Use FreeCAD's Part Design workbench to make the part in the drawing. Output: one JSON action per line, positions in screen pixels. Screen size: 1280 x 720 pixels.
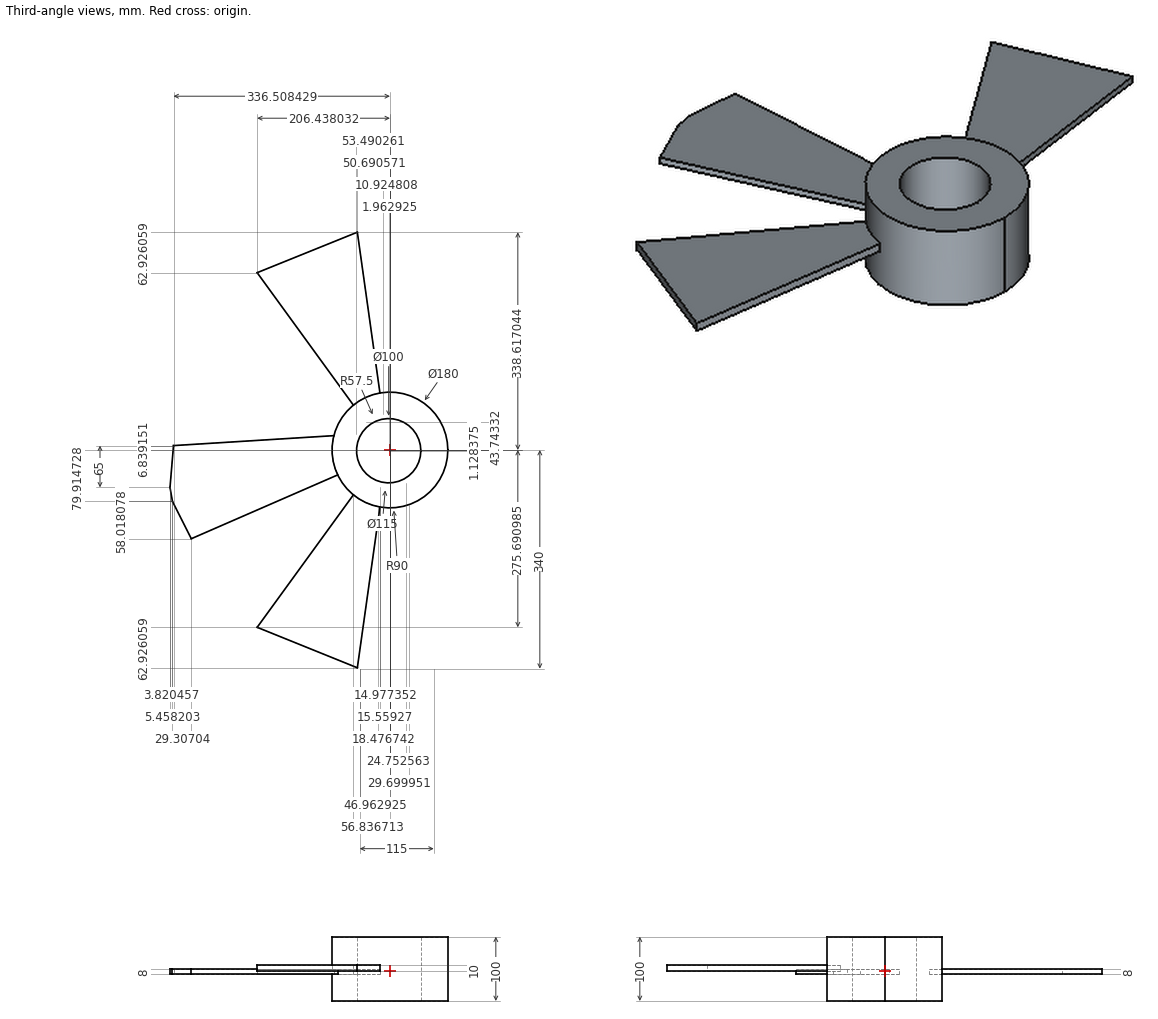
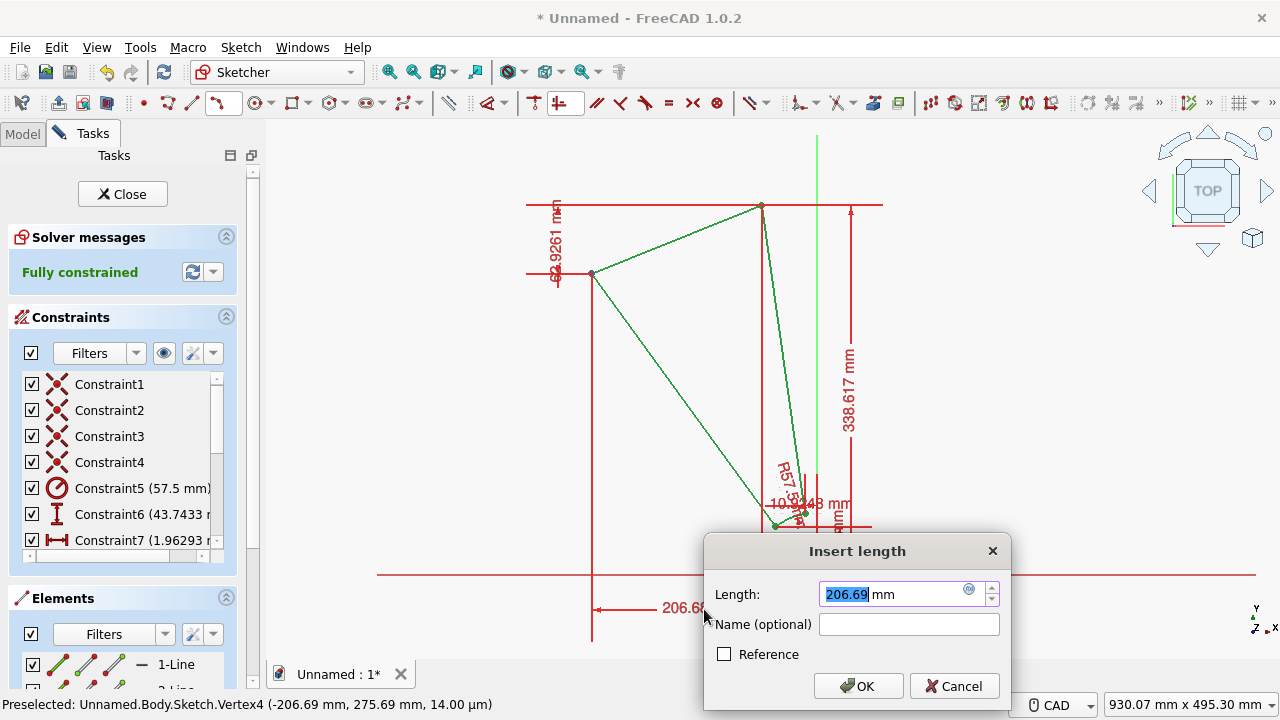
{"action": "type", "text": "206.438032"}
{"action": "key", "text": "Return"}
{"action": "key", "text": "Escape"}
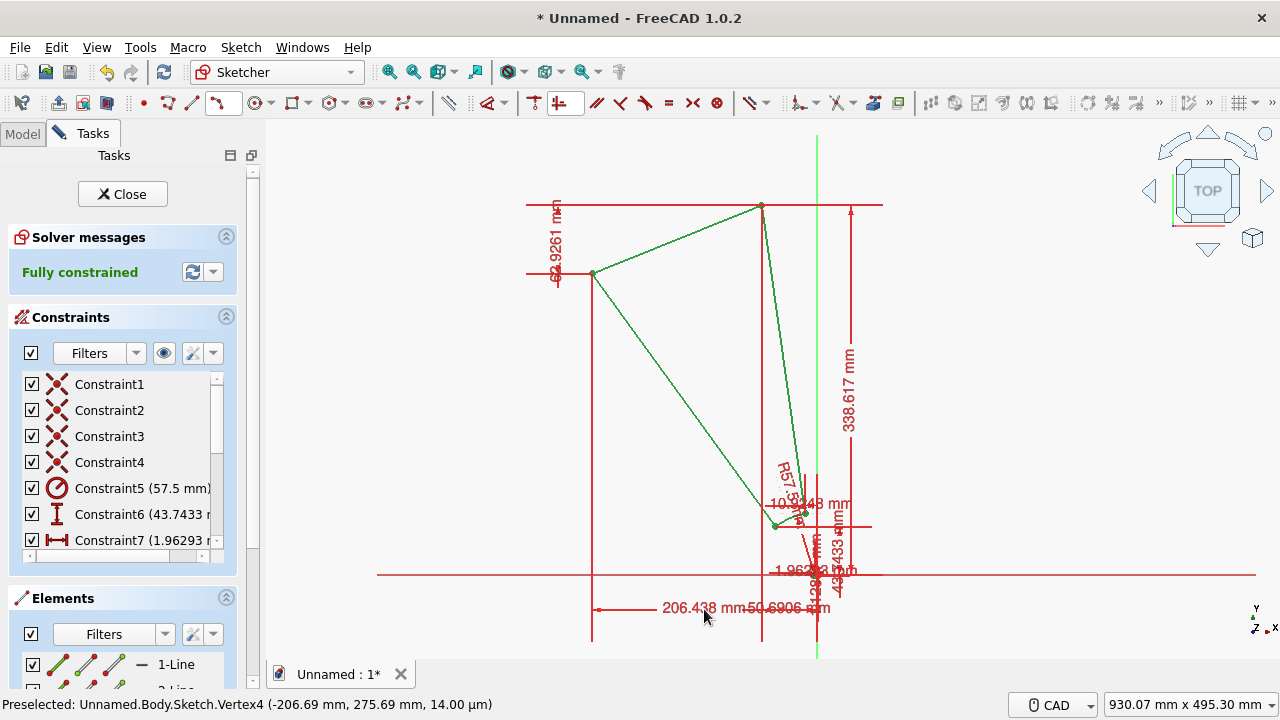
{"action": "left_click", "coordinate": [123, 194]}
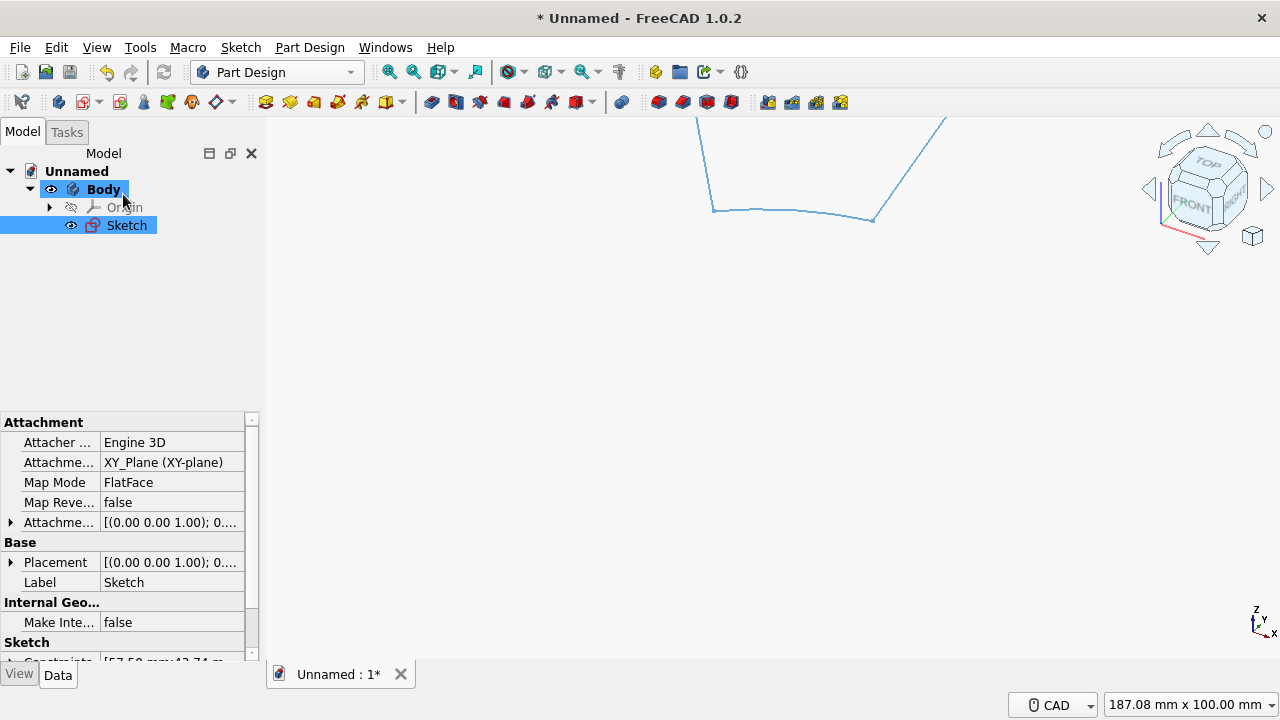
{"action": "left_click", "coordinate": [266, 102]}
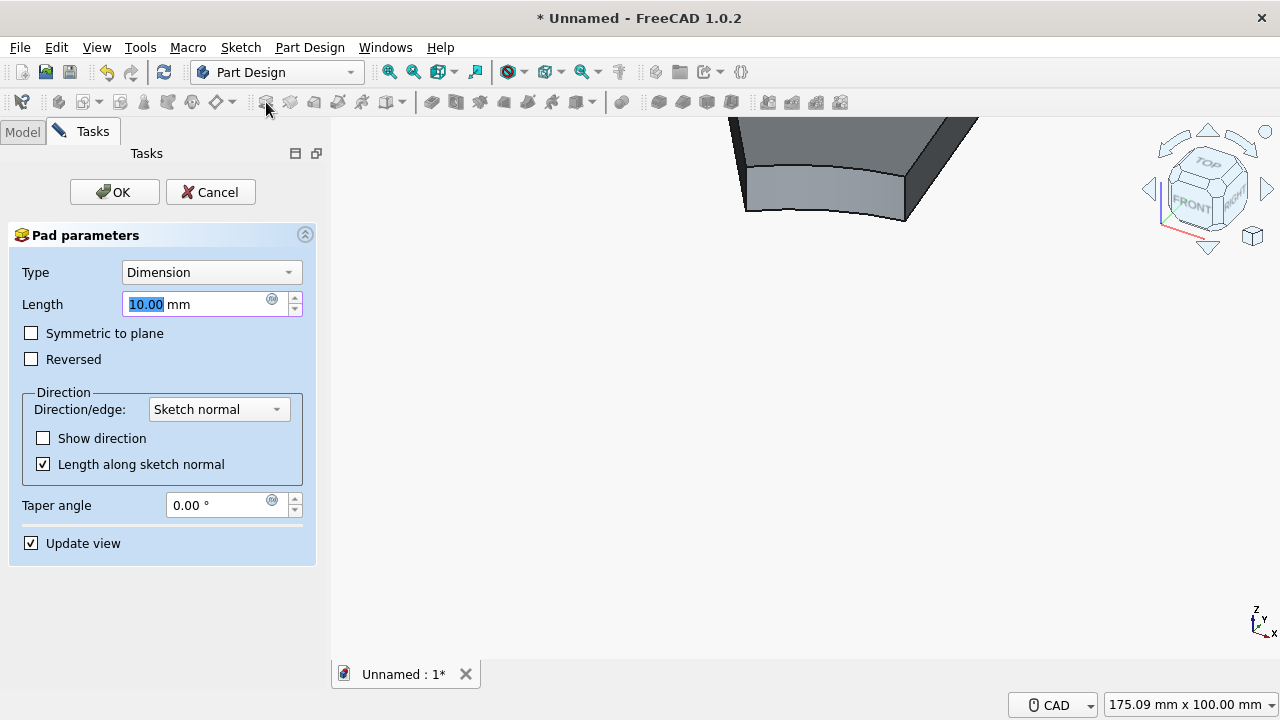
{"action": "type", "text": "8"}
{"action": "key", "text": "Tab"}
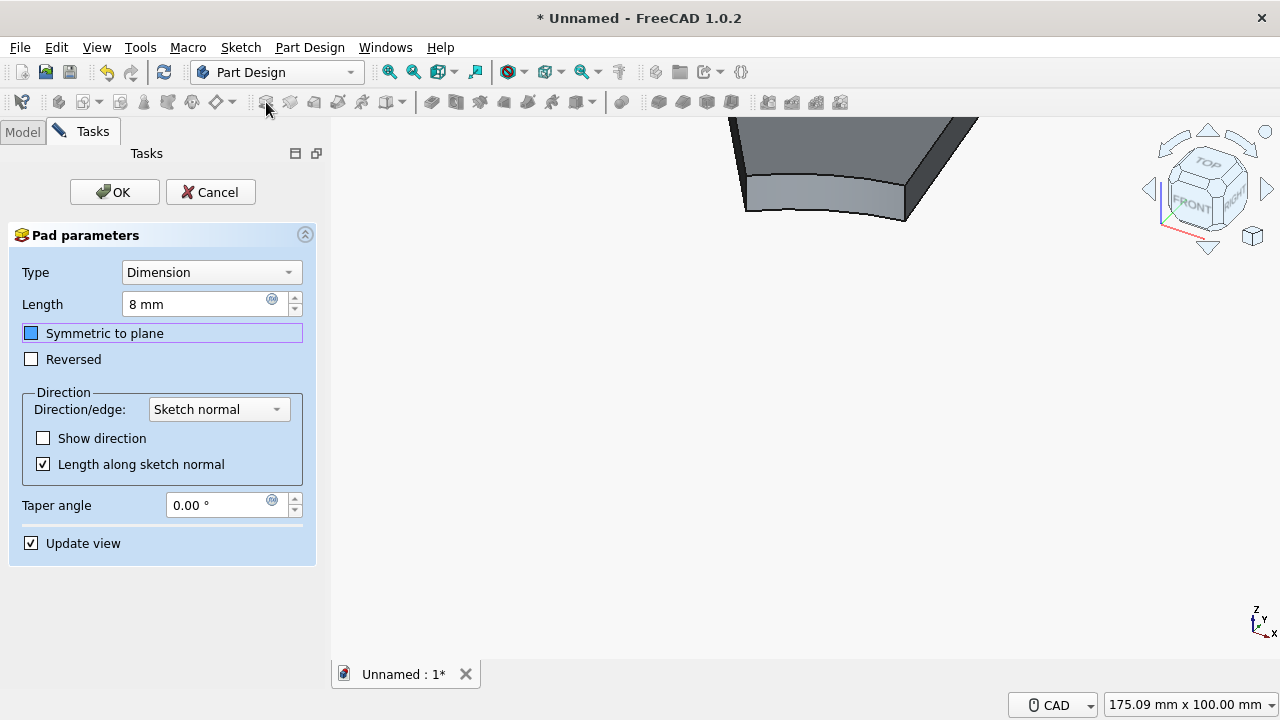
{"action": "left_click", "coordinate": [30, 333]}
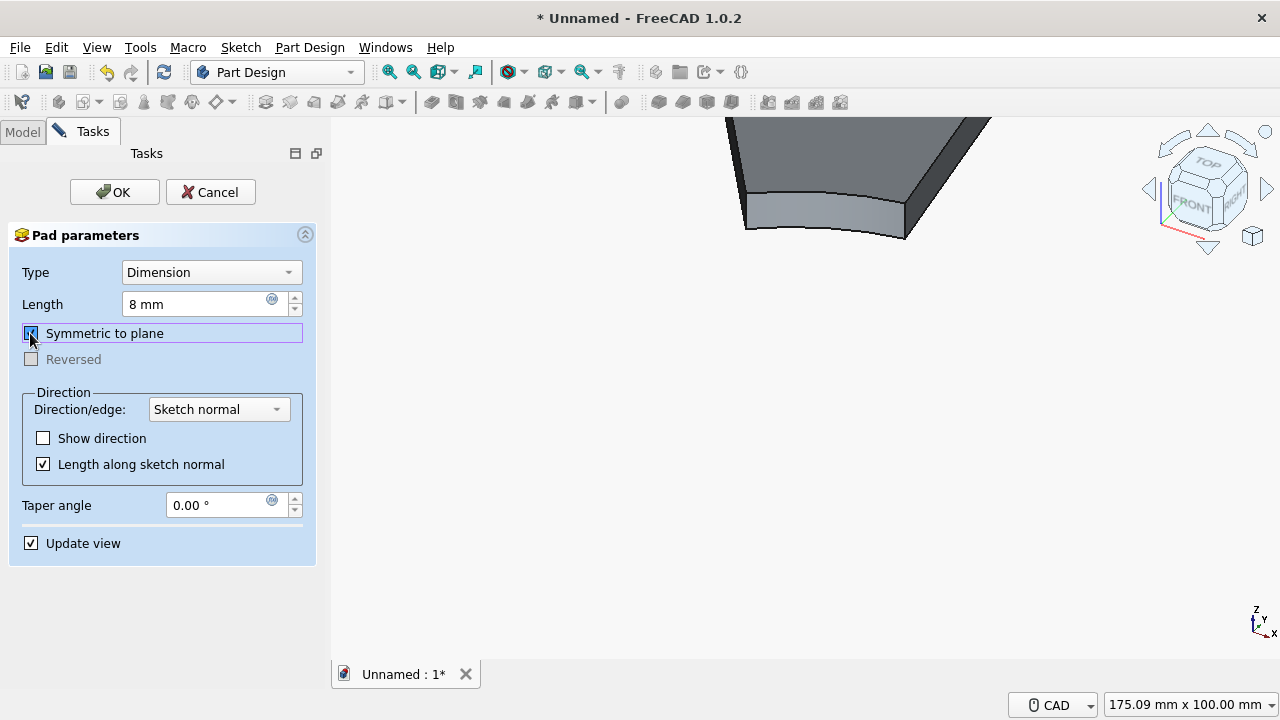
{"action": "left_click", "coordinate": [115, 192]}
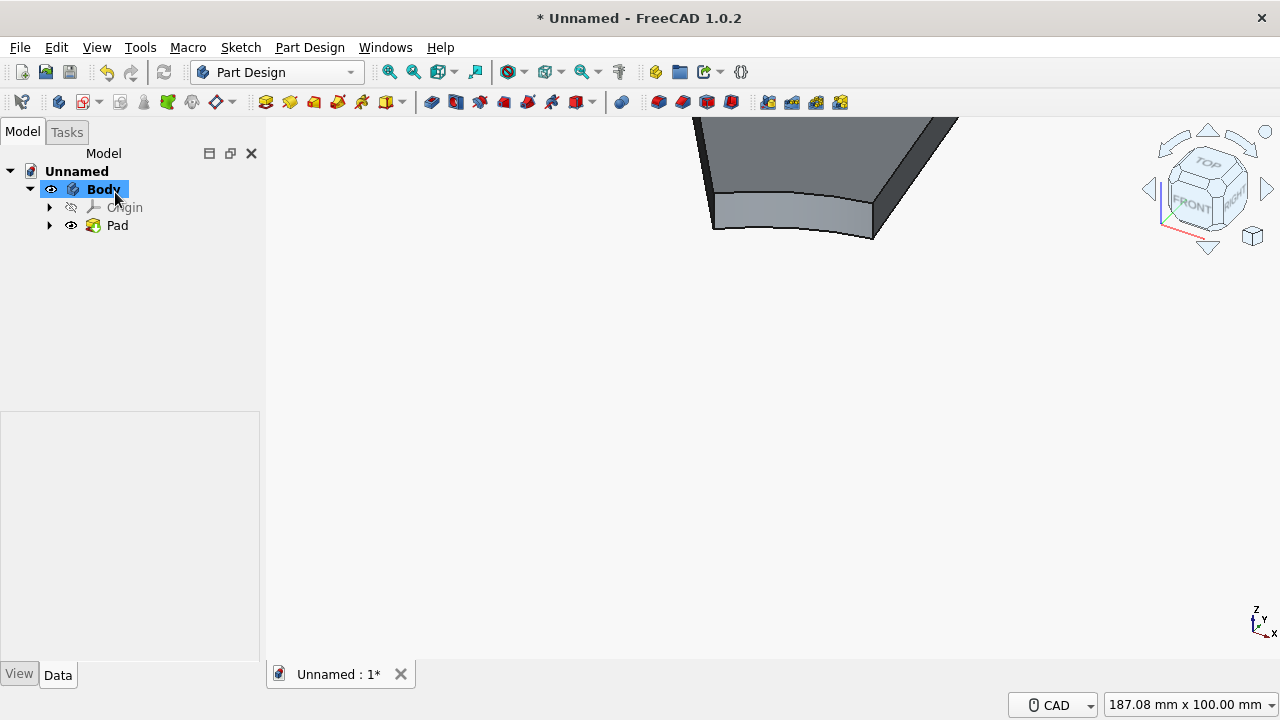
{"action": "left_click", "coordinate": [390, 72]}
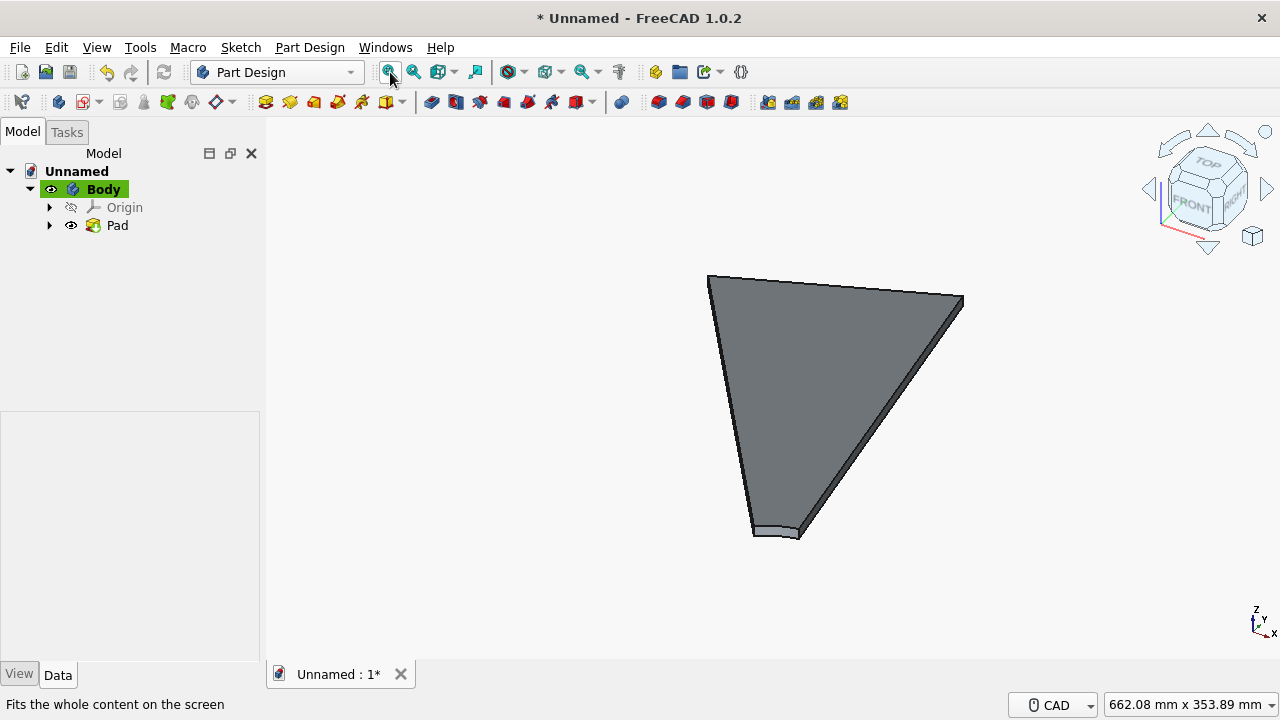
{"action": "left_click", "coordinate": [60, 102]}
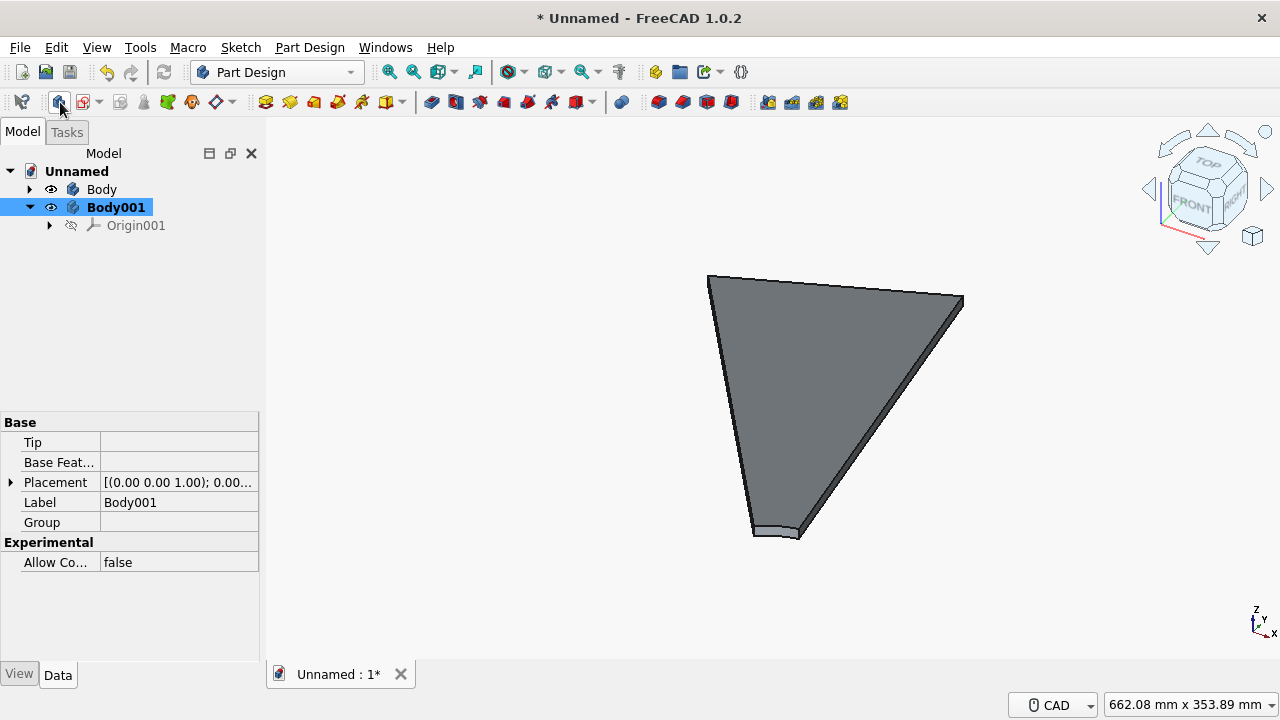
{"action": "left_click", "coordinate": [306, 619]}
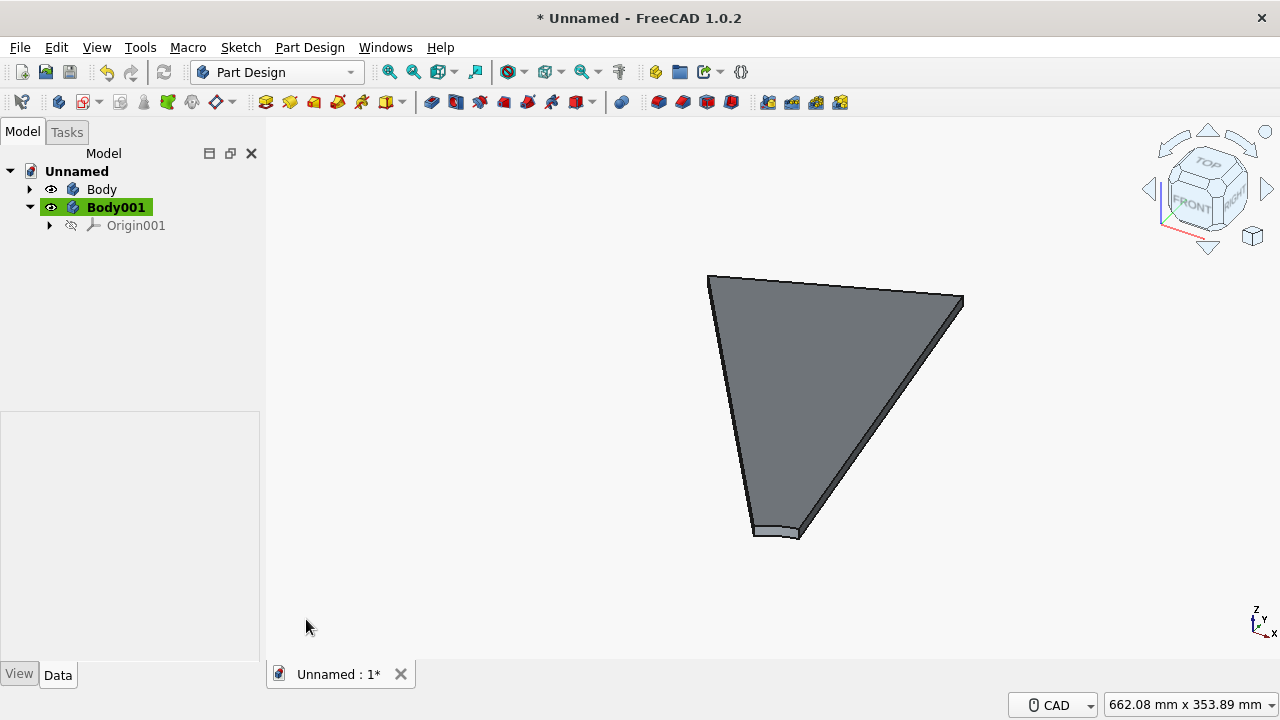
{"action": "left_click", "coordinate": [84, 102]}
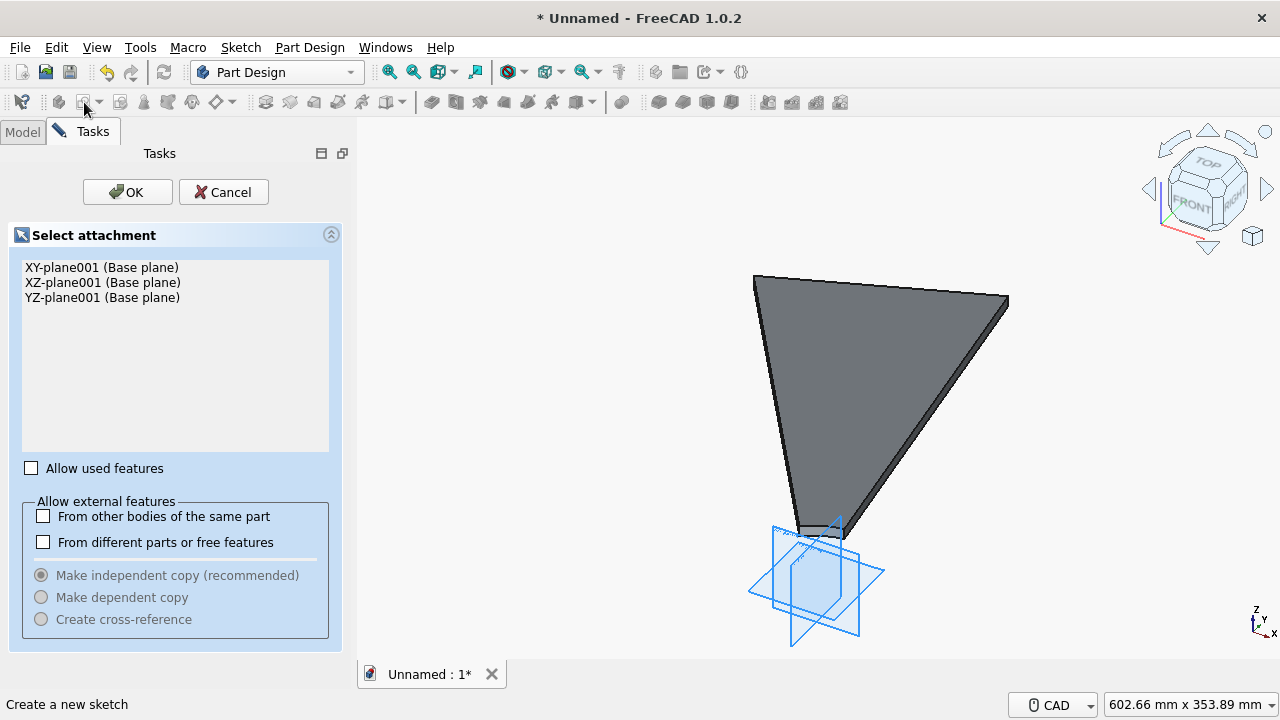
{"action": "left_click", "coordinate": [82, 268]}